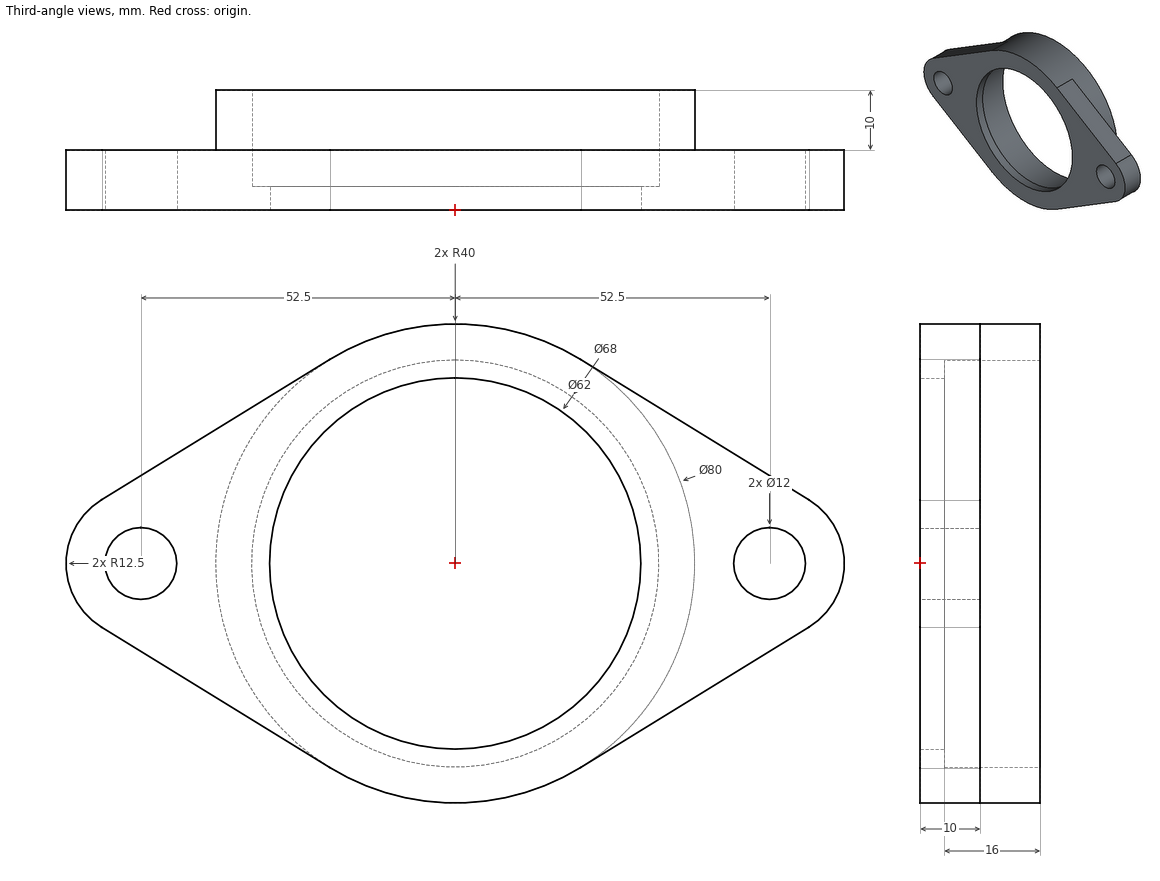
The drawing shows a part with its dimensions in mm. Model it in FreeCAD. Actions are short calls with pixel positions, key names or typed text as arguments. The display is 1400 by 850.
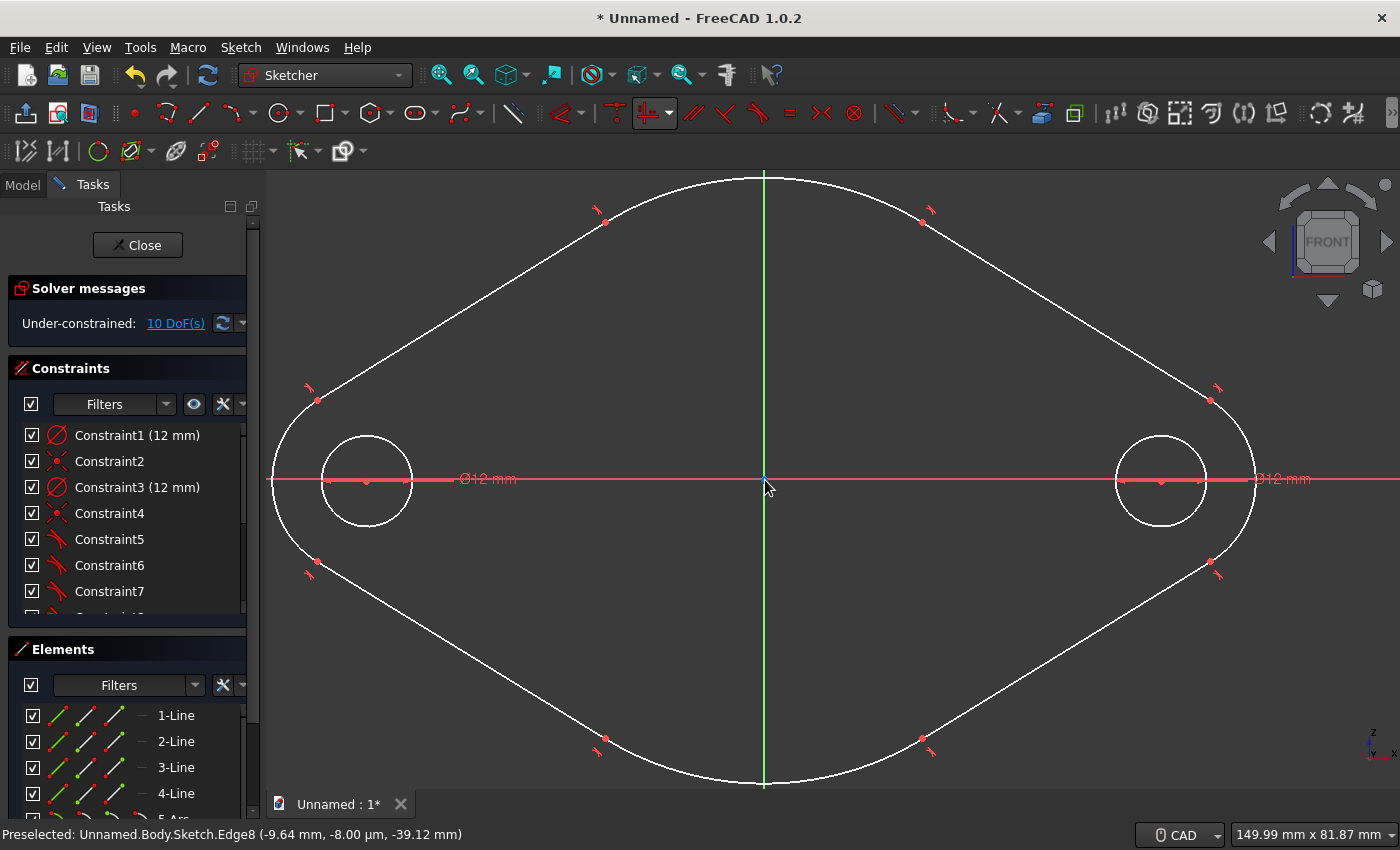
drag(754, 469, 774, 490)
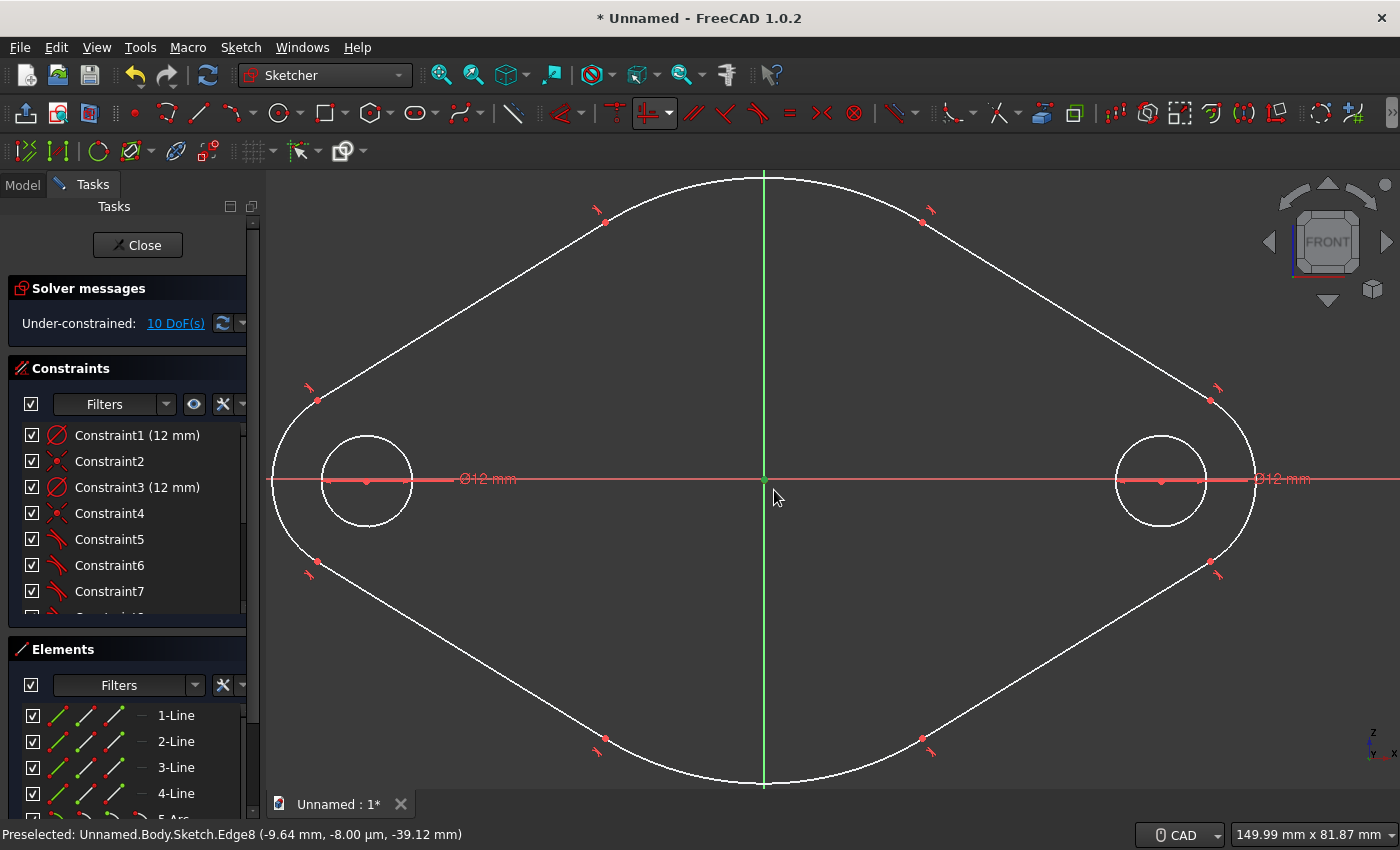
click(616, 114)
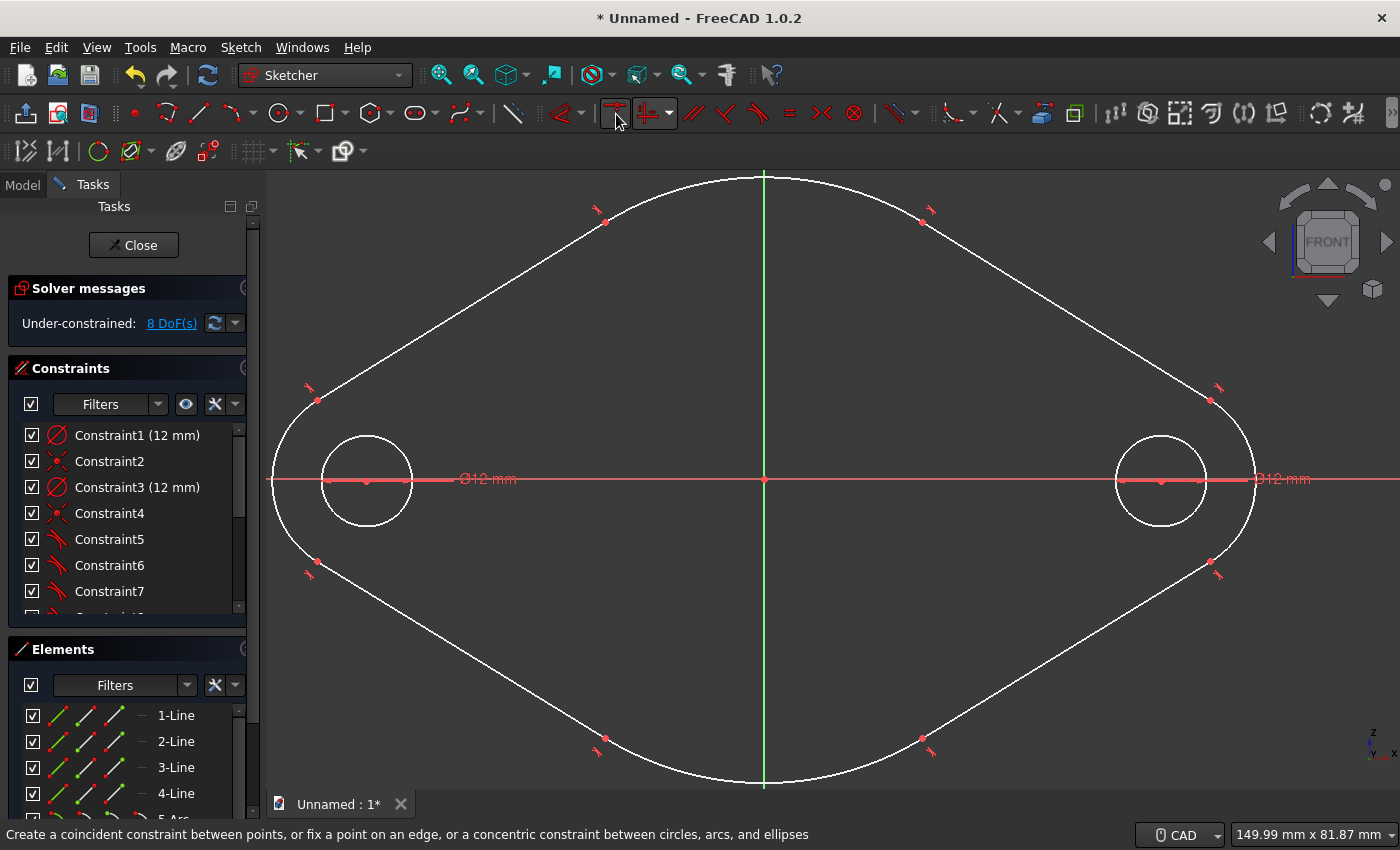
scroll(765, 480, down, 2)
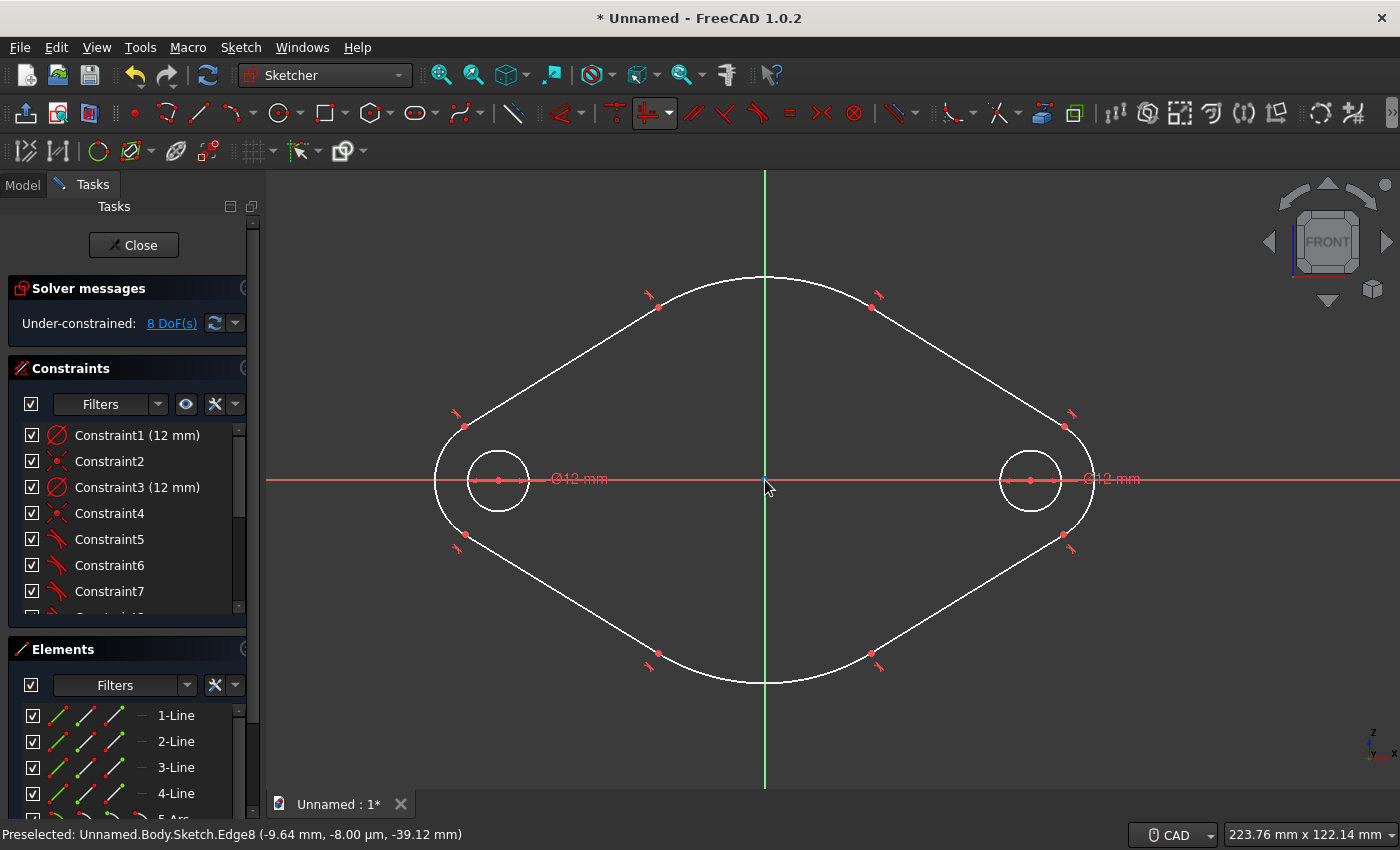
click(440, 456)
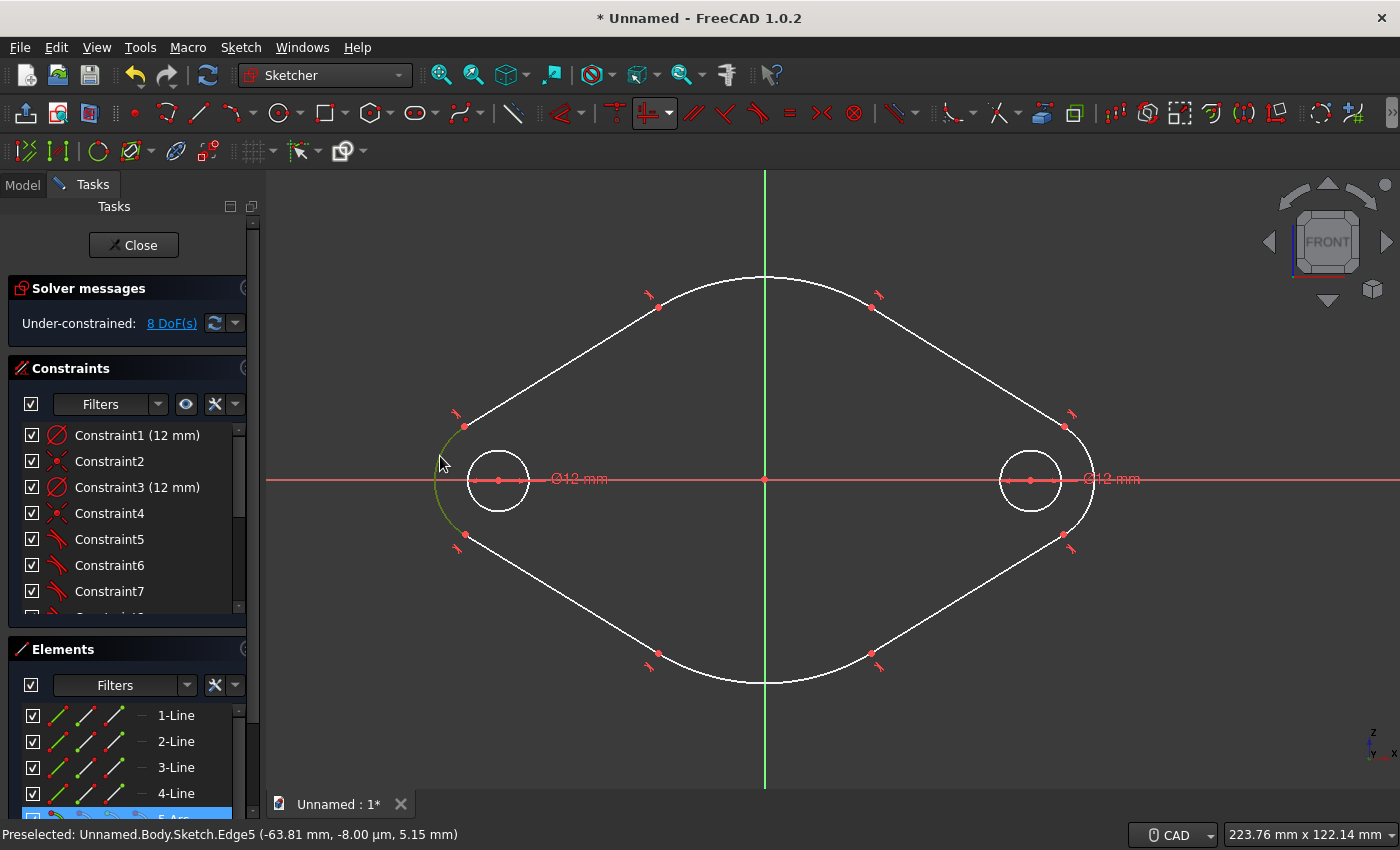
click(1089, 506)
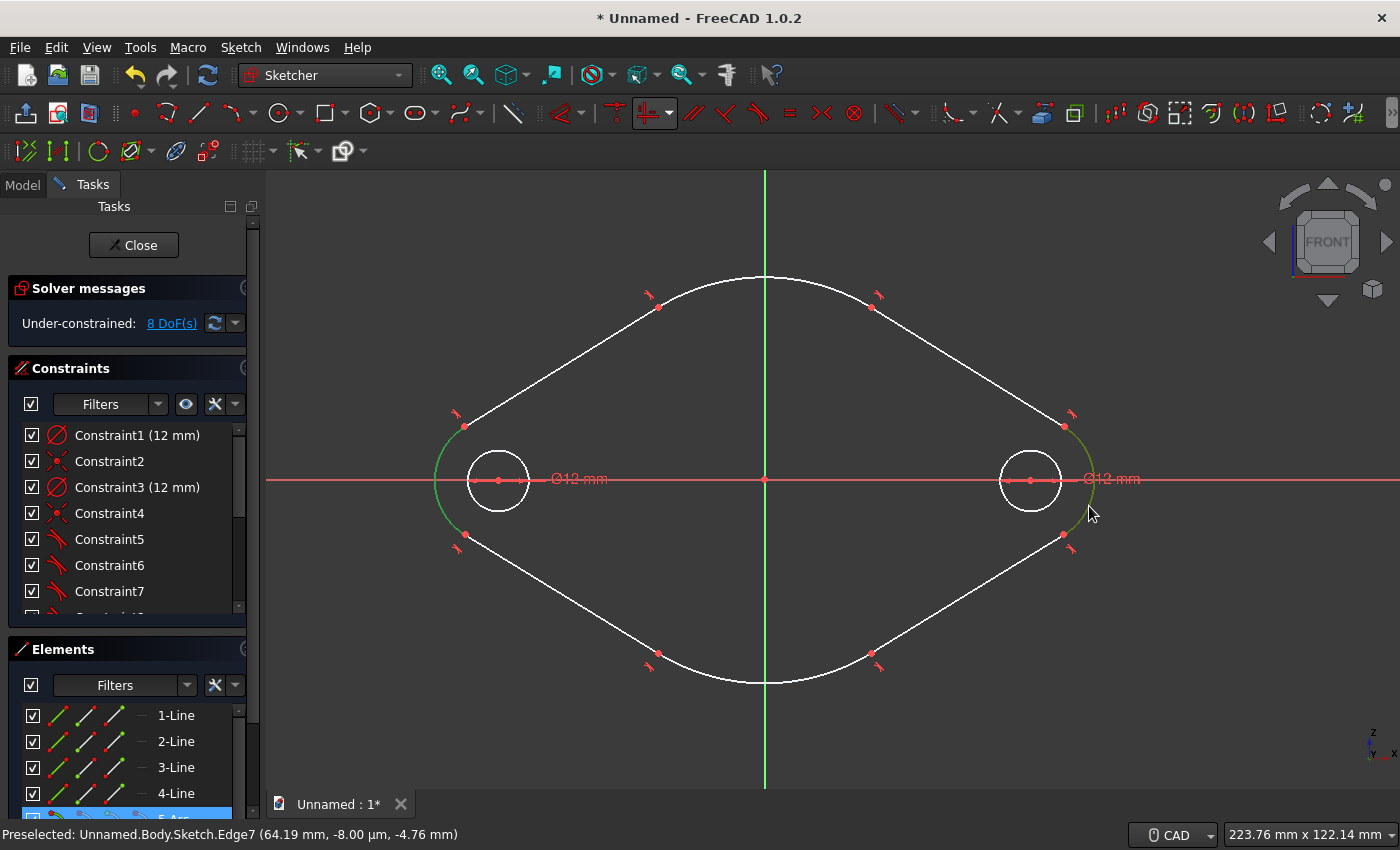
click(790, 114)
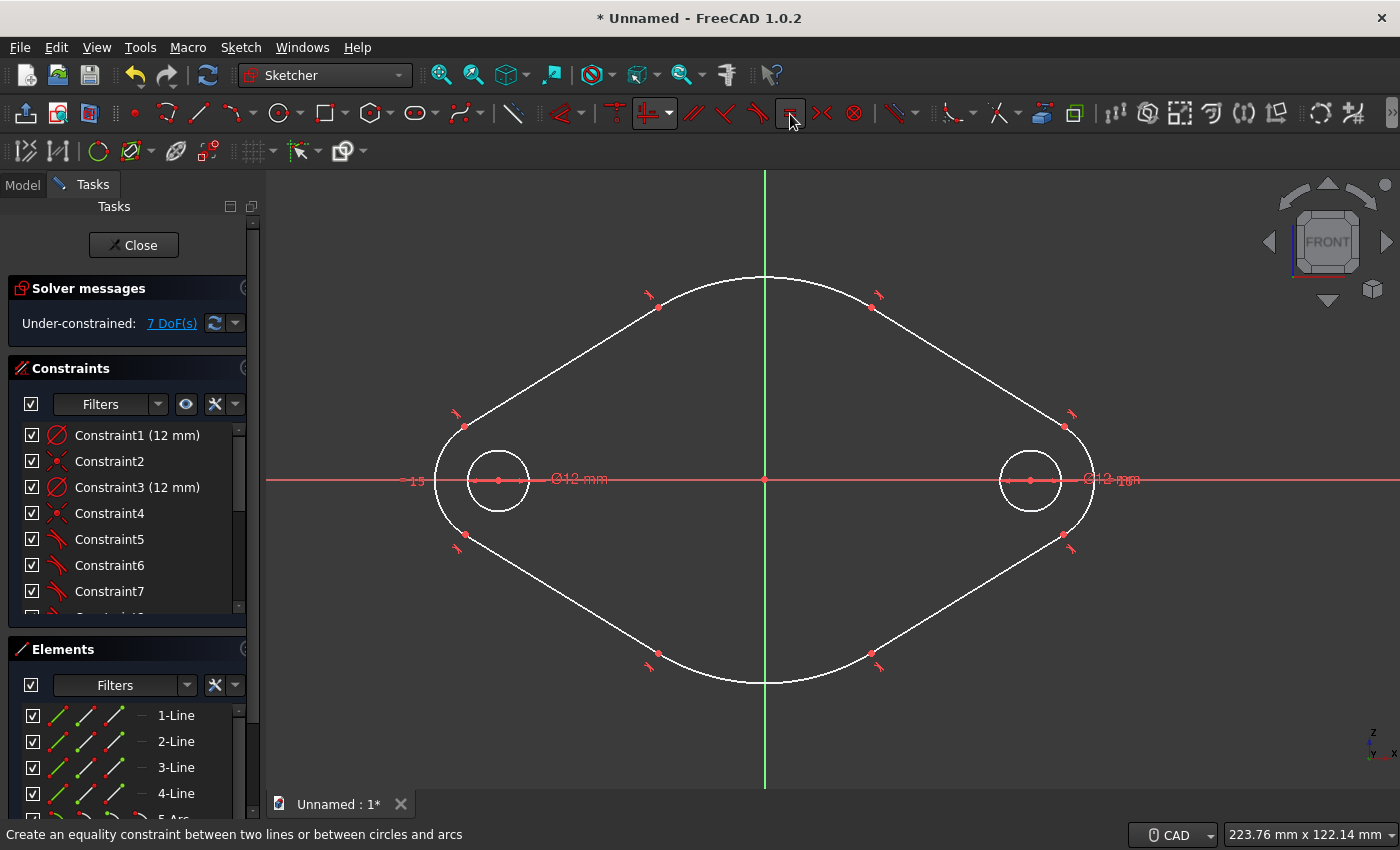
click(809, 282)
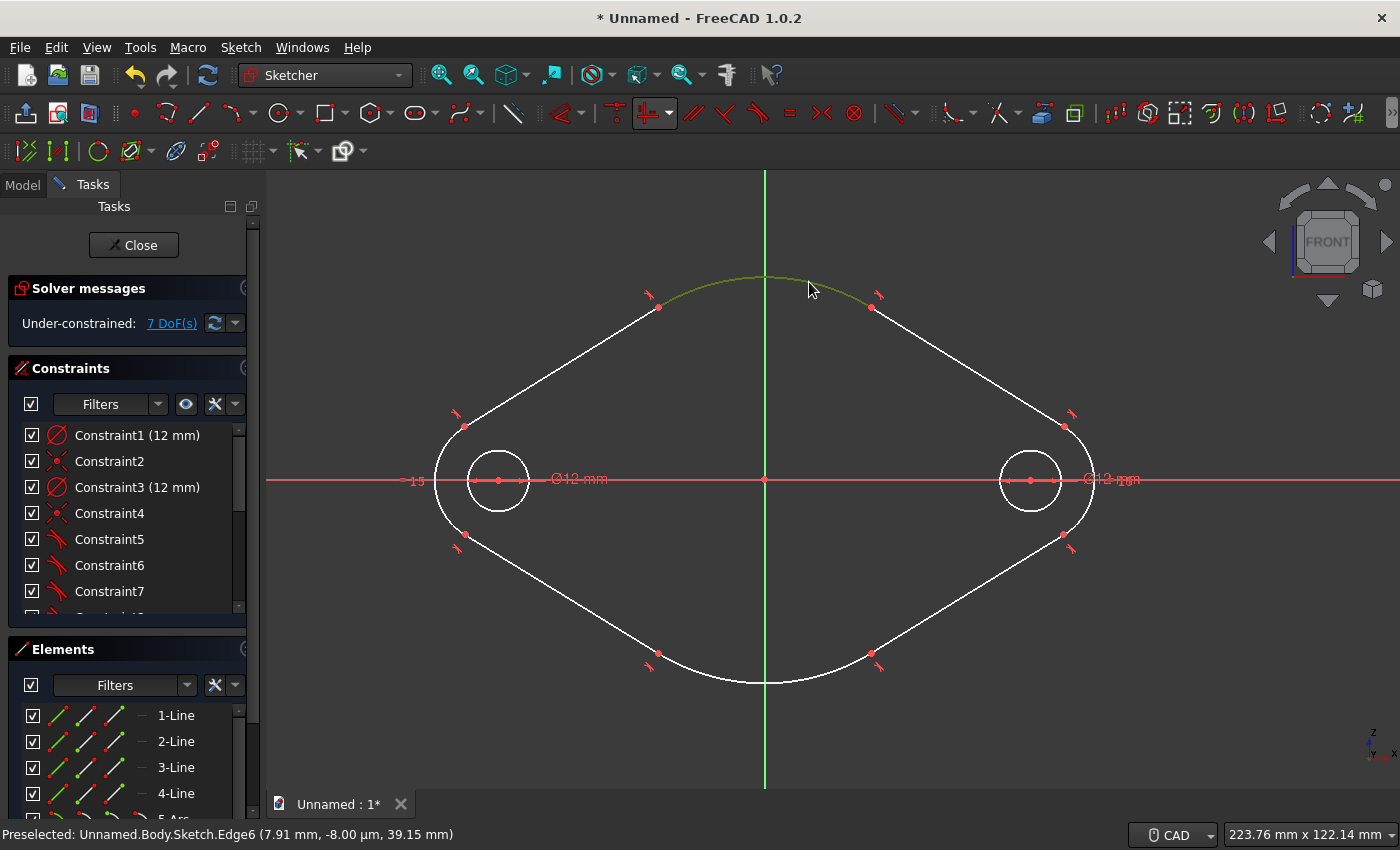
click(720, 678)